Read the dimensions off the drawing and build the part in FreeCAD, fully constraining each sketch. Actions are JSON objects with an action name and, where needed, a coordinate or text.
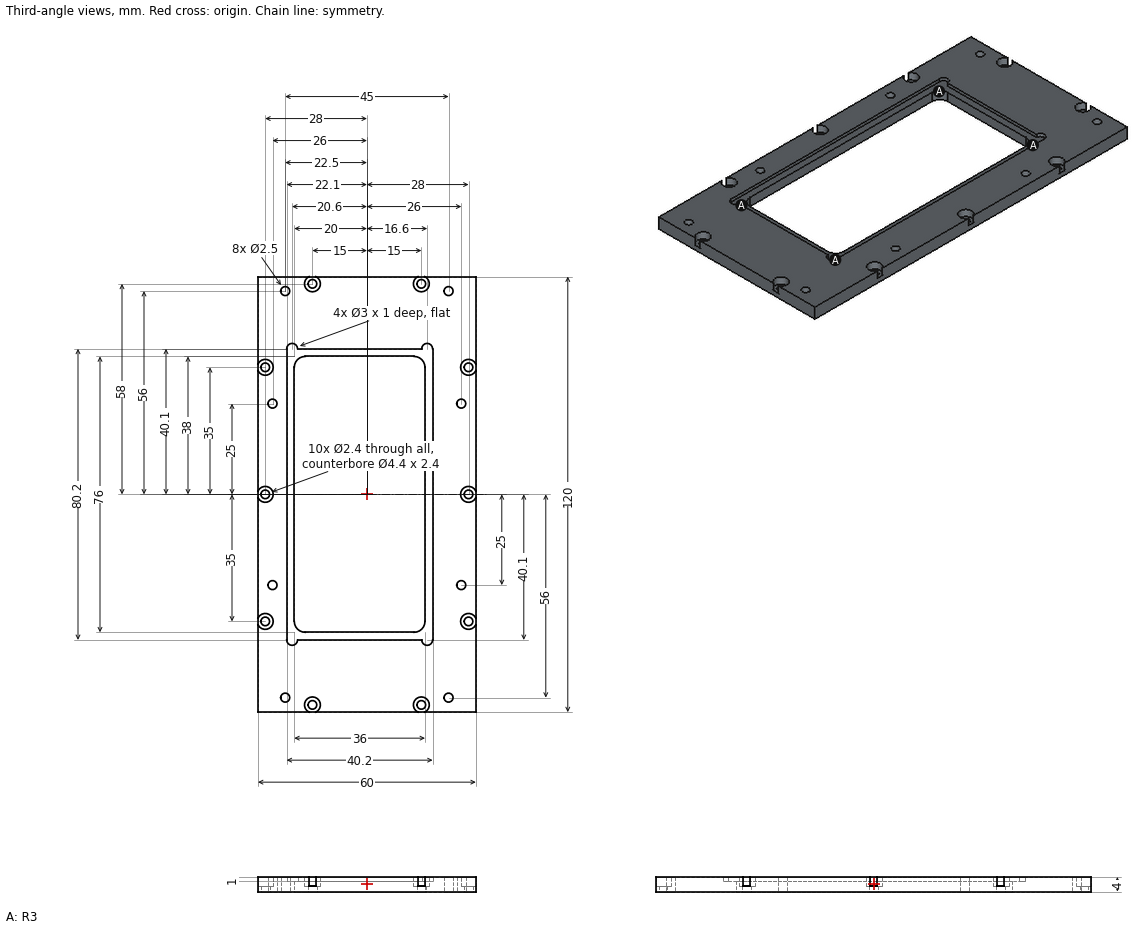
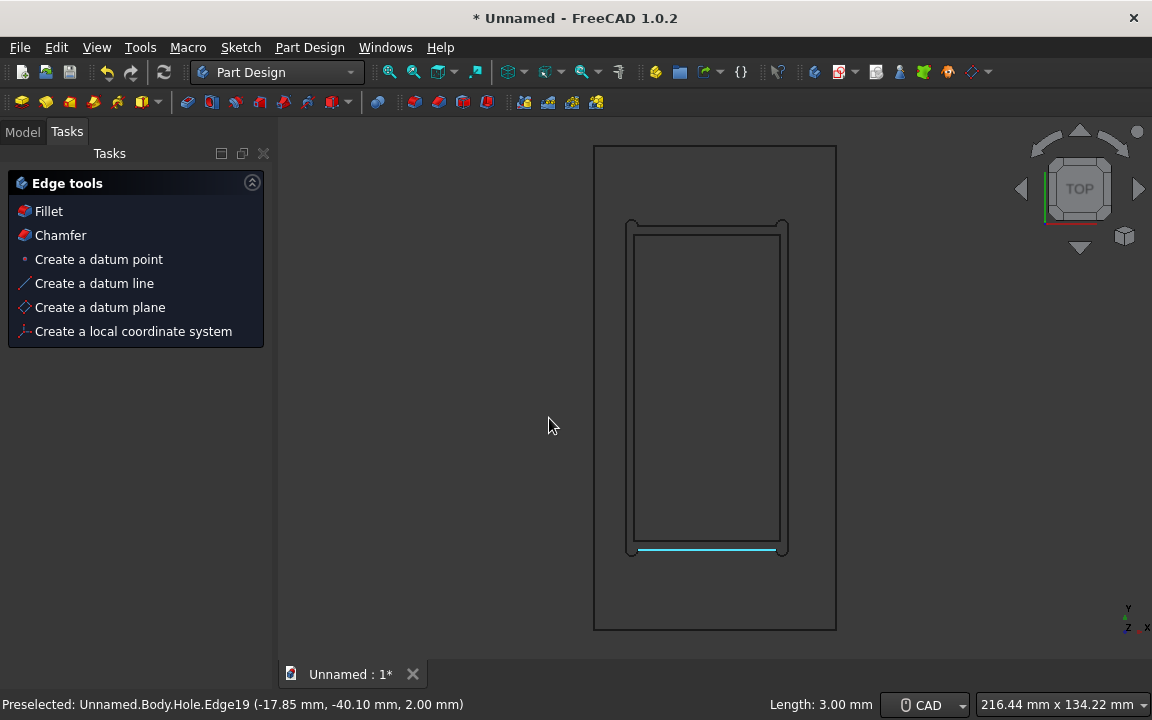
{"action": "scroll", "coordinate": [634, 540], "scroll_direction": "up", "scroll_amount": 6}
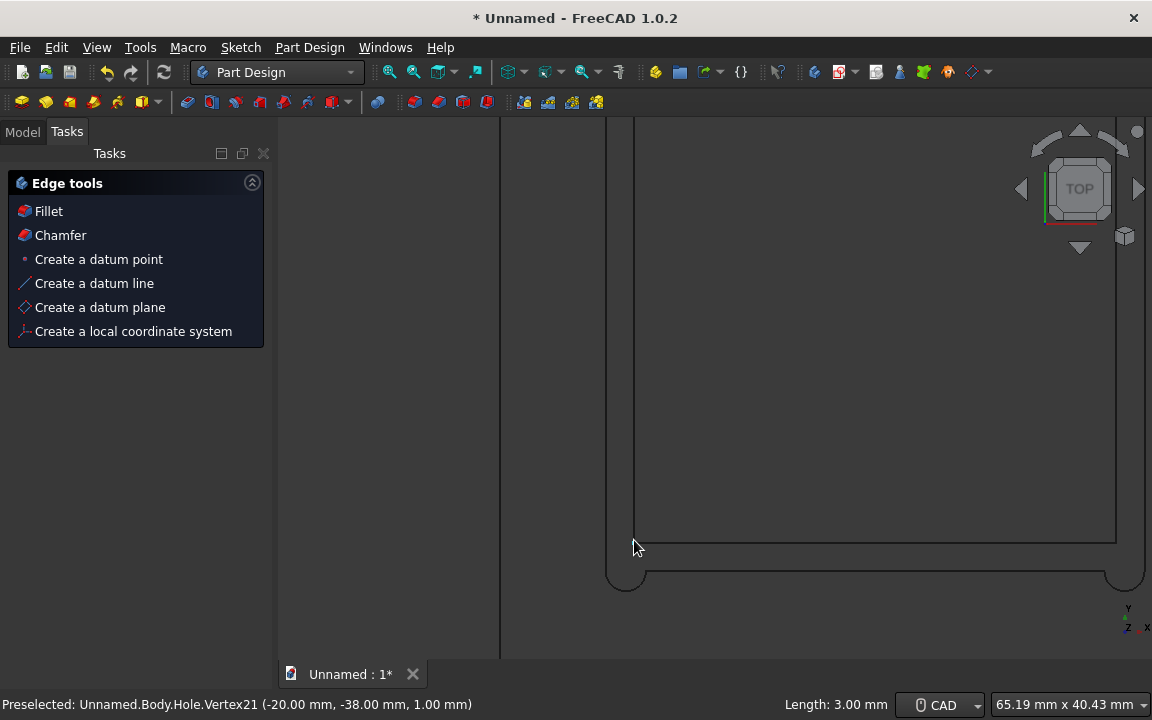
{"action": "key", "text": "v f"}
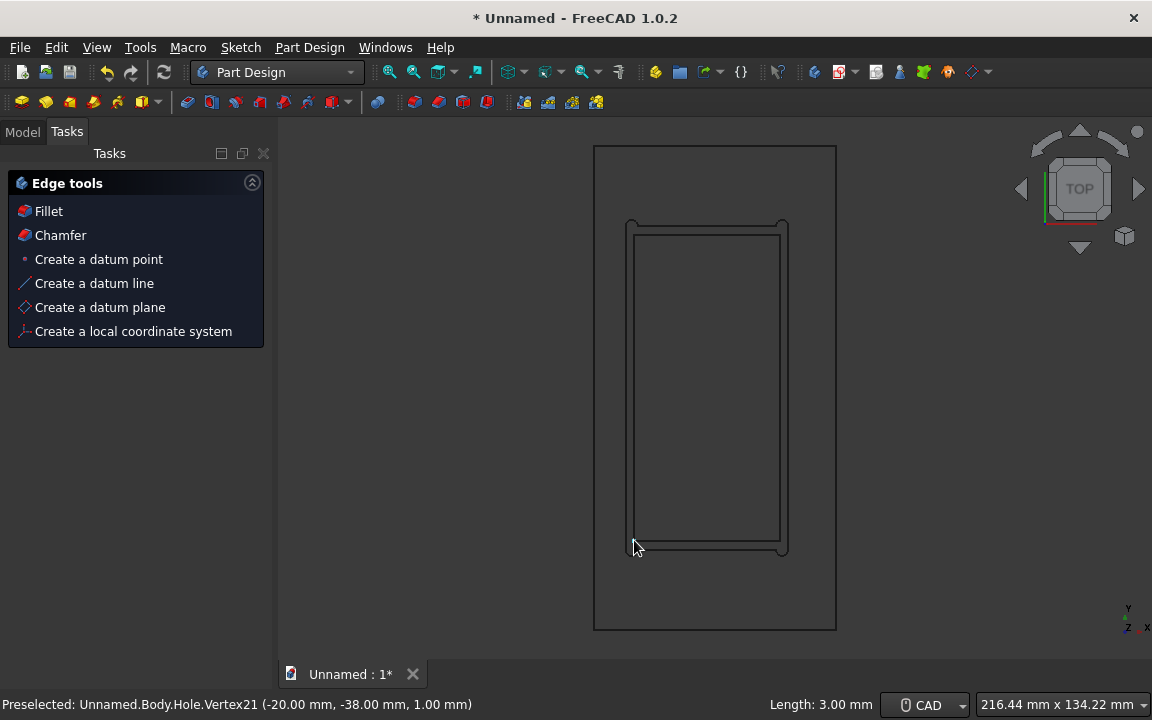
{"action": "key", "text": "1"}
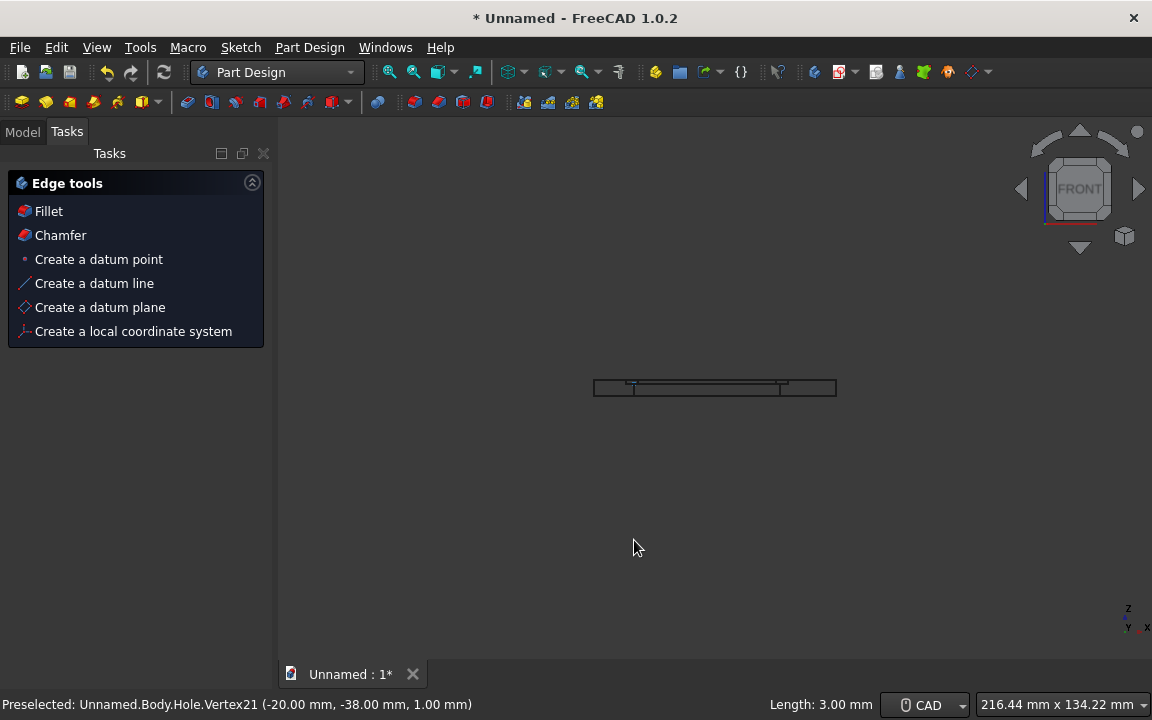
{"action": "key", "text": "v f"}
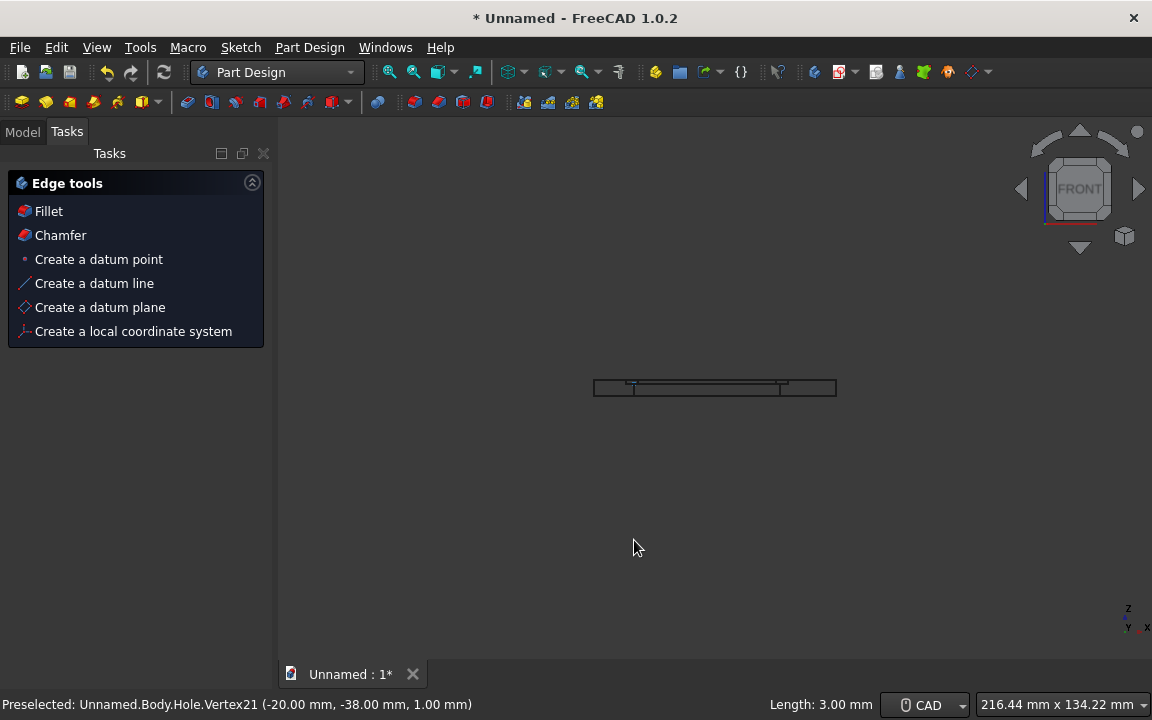
{"action": "left_click", "coordinate": [634, 389], "text": "ctrl"}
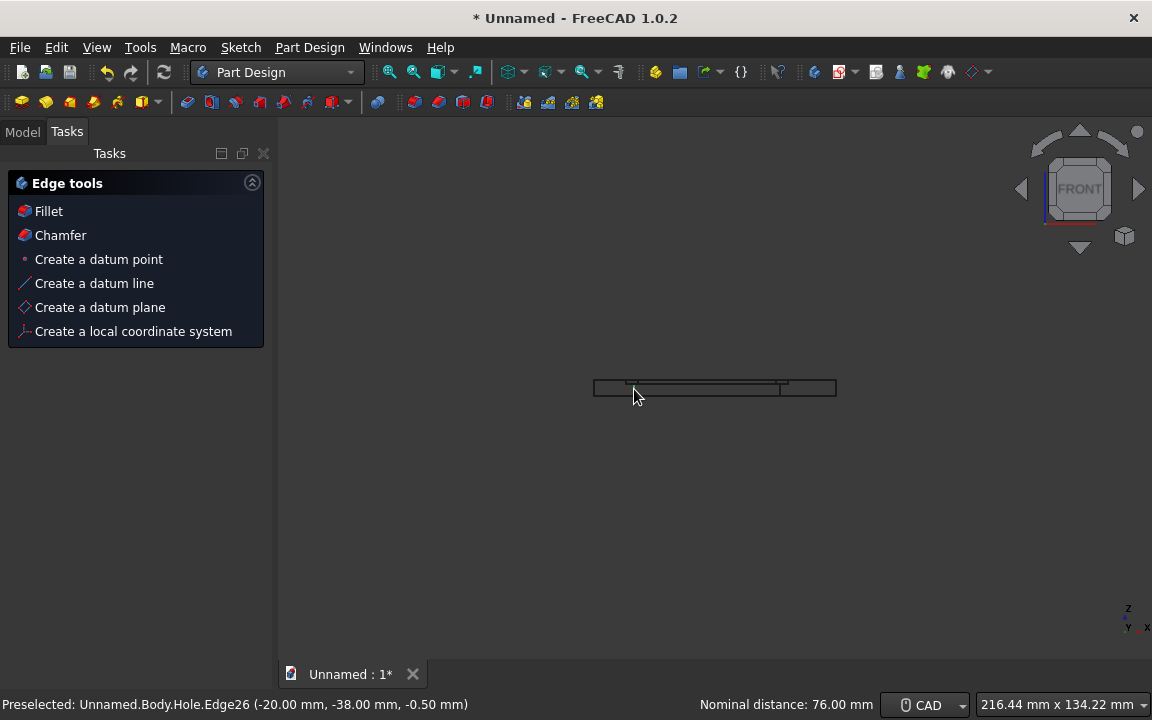
{"action": "left_click", "coordinate": [780, 389], "text": "ctrl"}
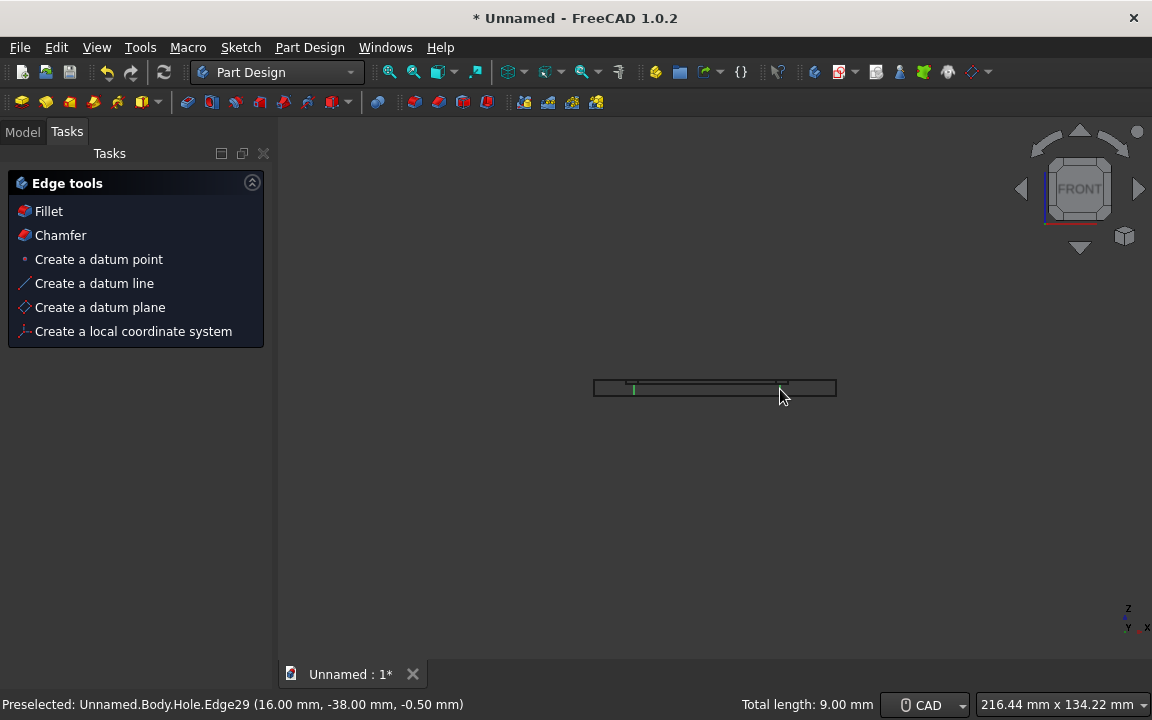
{"action": "scroll", "coordinate": [780, 389], "scroll_direction": "up", "scroll_amount": 6}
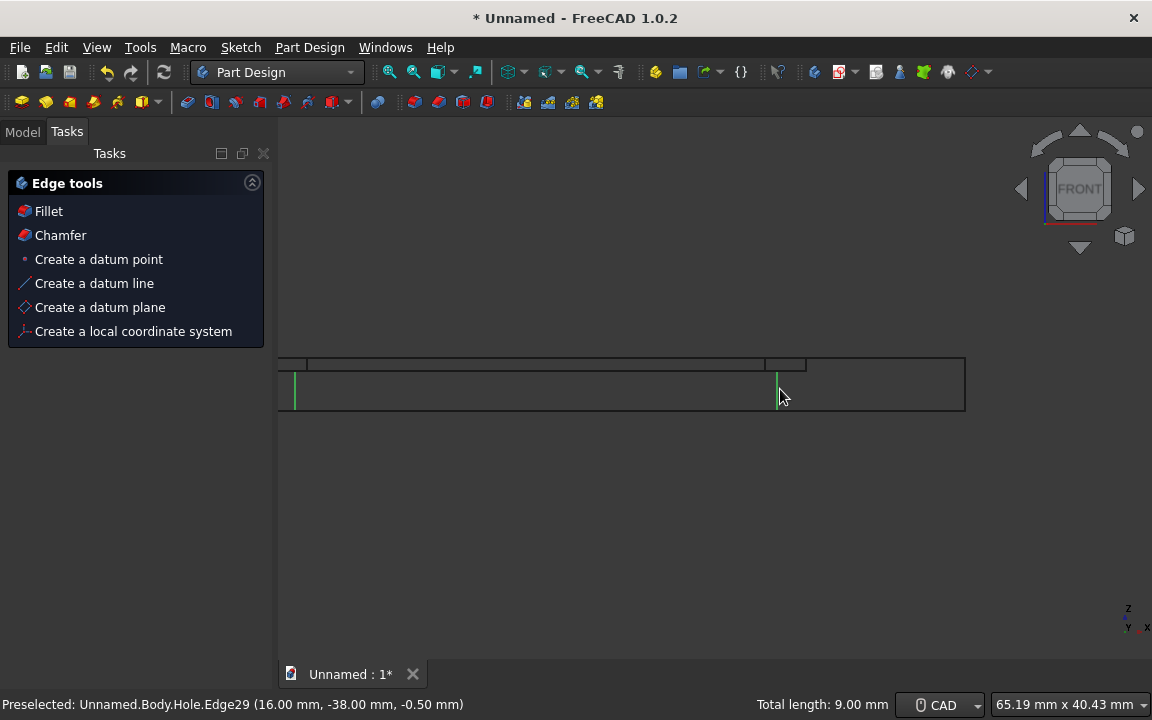
{"action": "key", "text": "v f"}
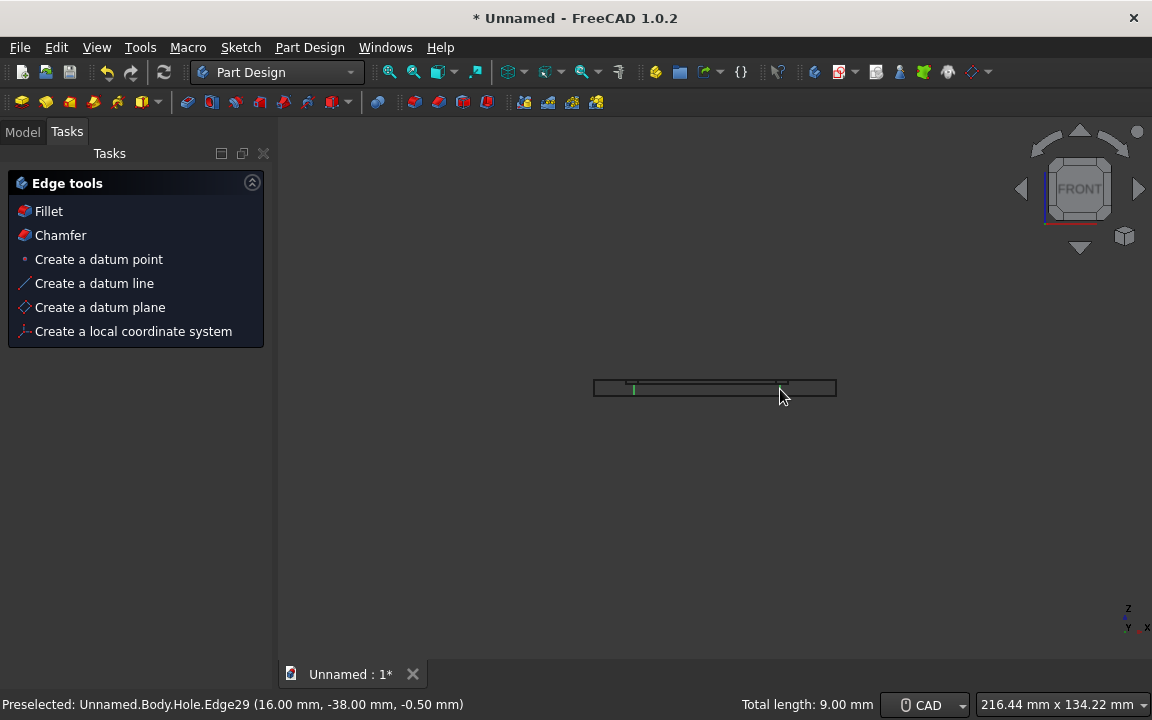
{"action": "key", "text": "3"}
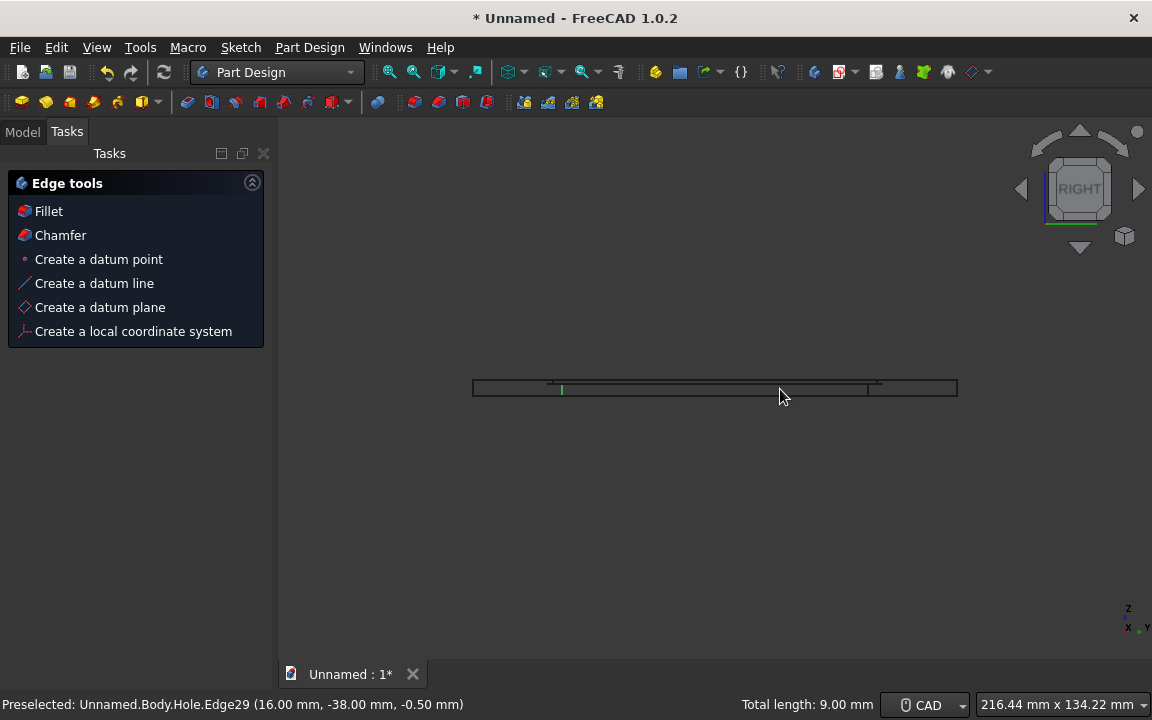
{"action": "left_click", "coordinate": [868, 389], "text": "ctrl"}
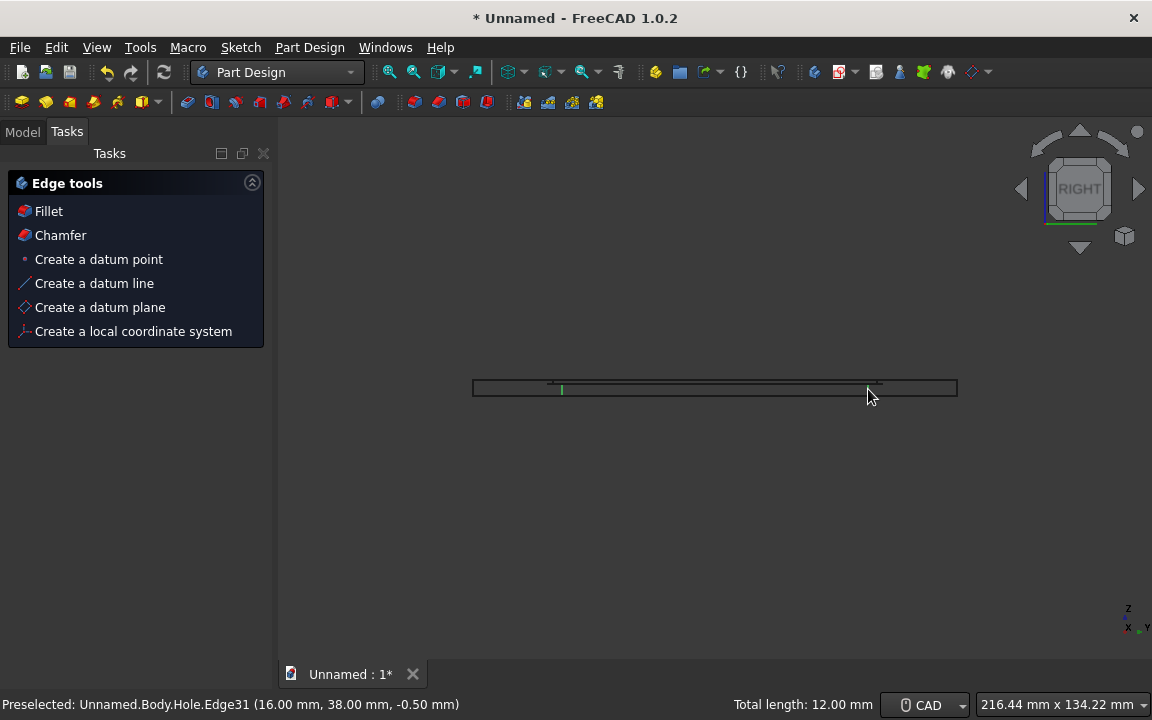
{"action": "key", "text": "v 1"}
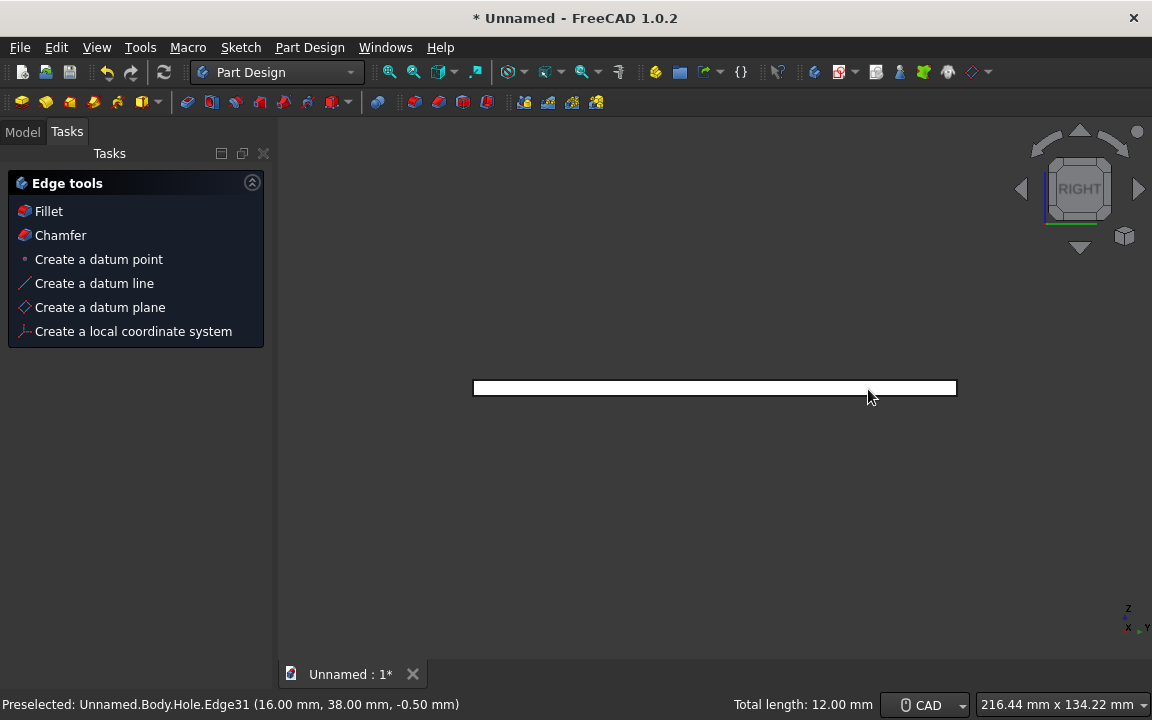
{"action": "left_click", "coordinate": [416, 102]}